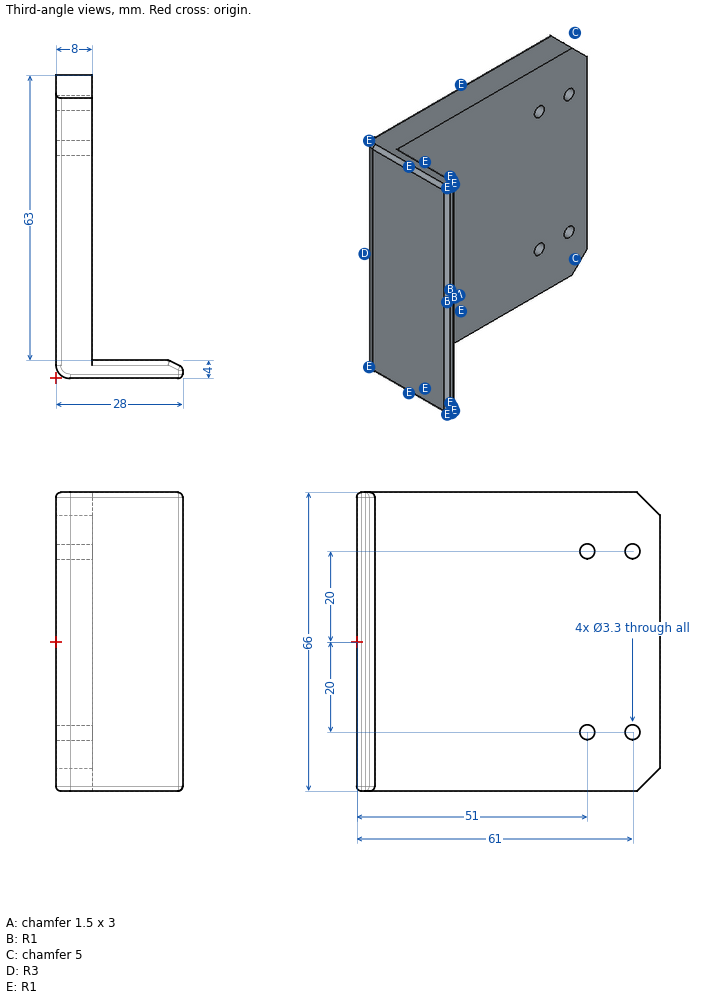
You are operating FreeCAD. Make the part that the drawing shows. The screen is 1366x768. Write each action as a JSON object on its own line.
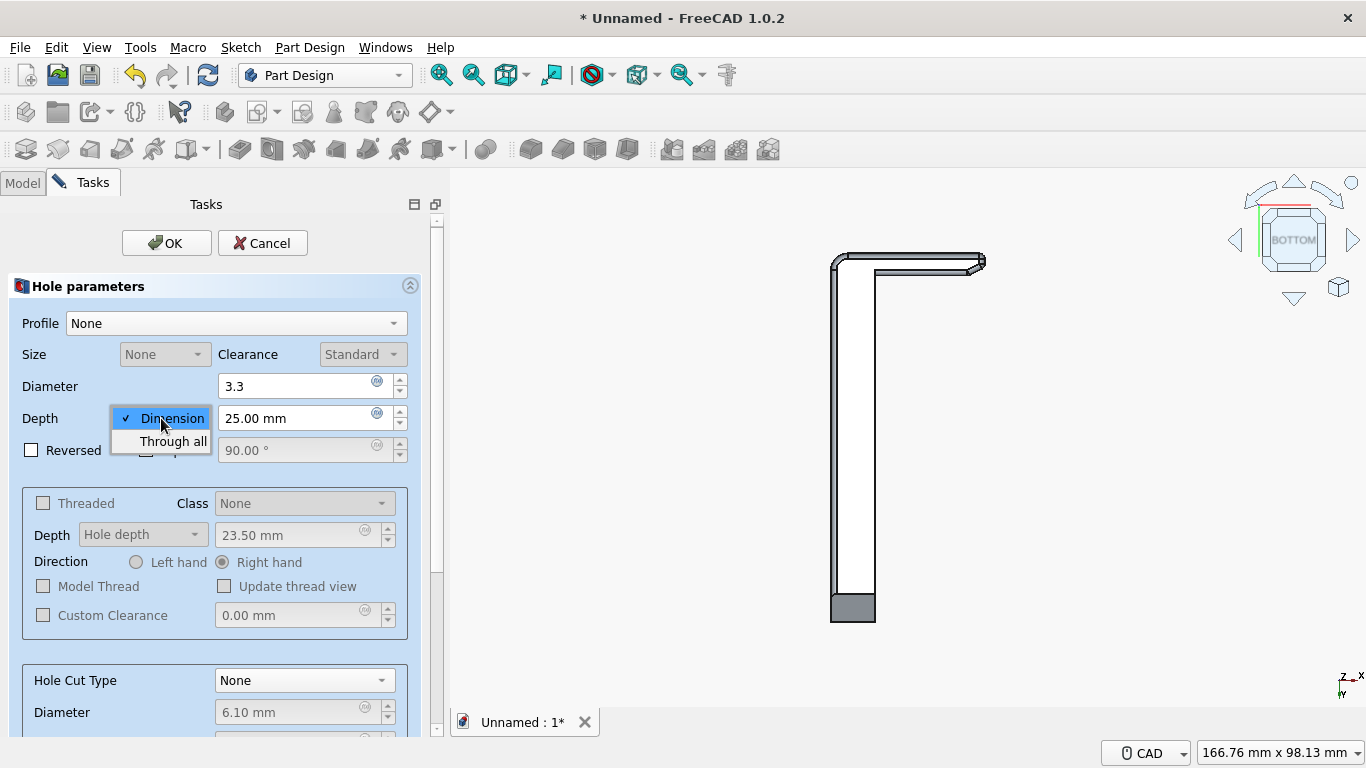
{"action": "left_click", "coordinate": [160, 442]}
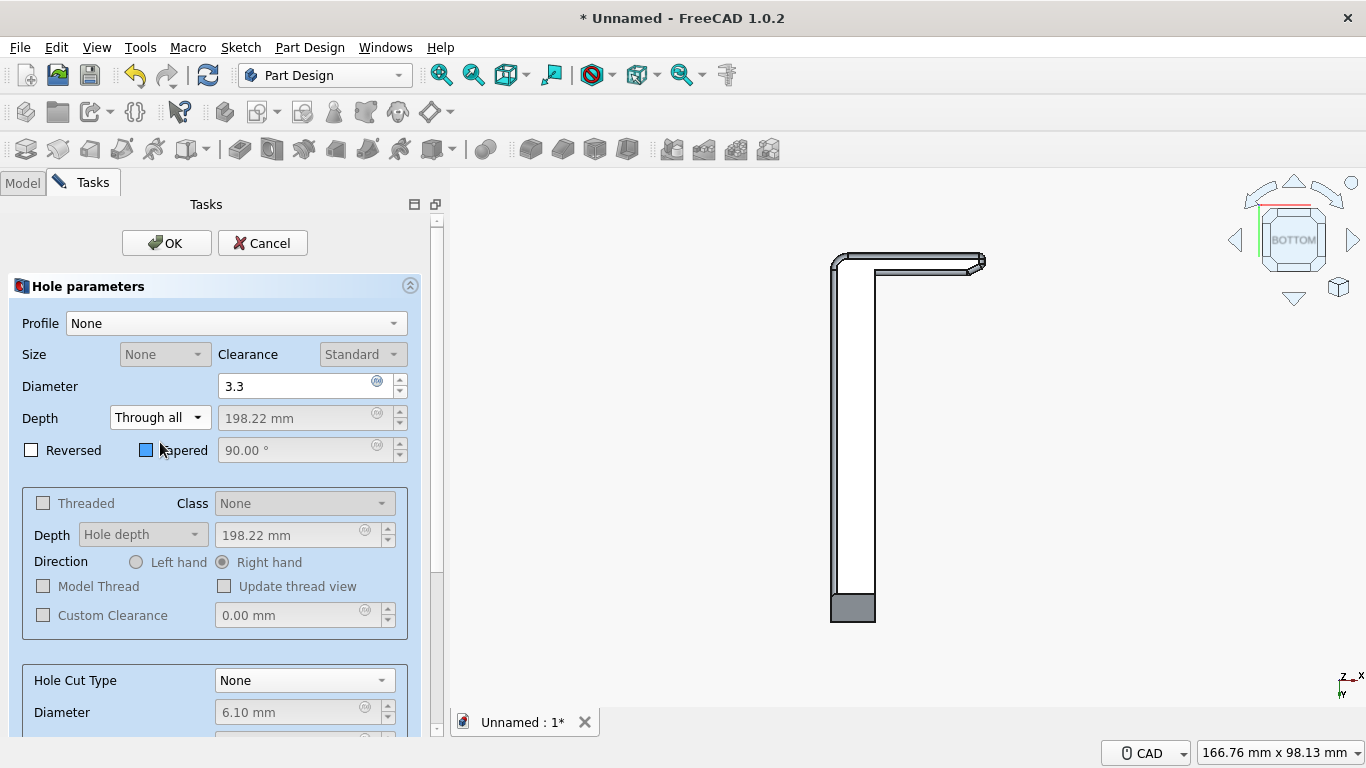
{"action": "left_click", "coordinate": [30, 450]}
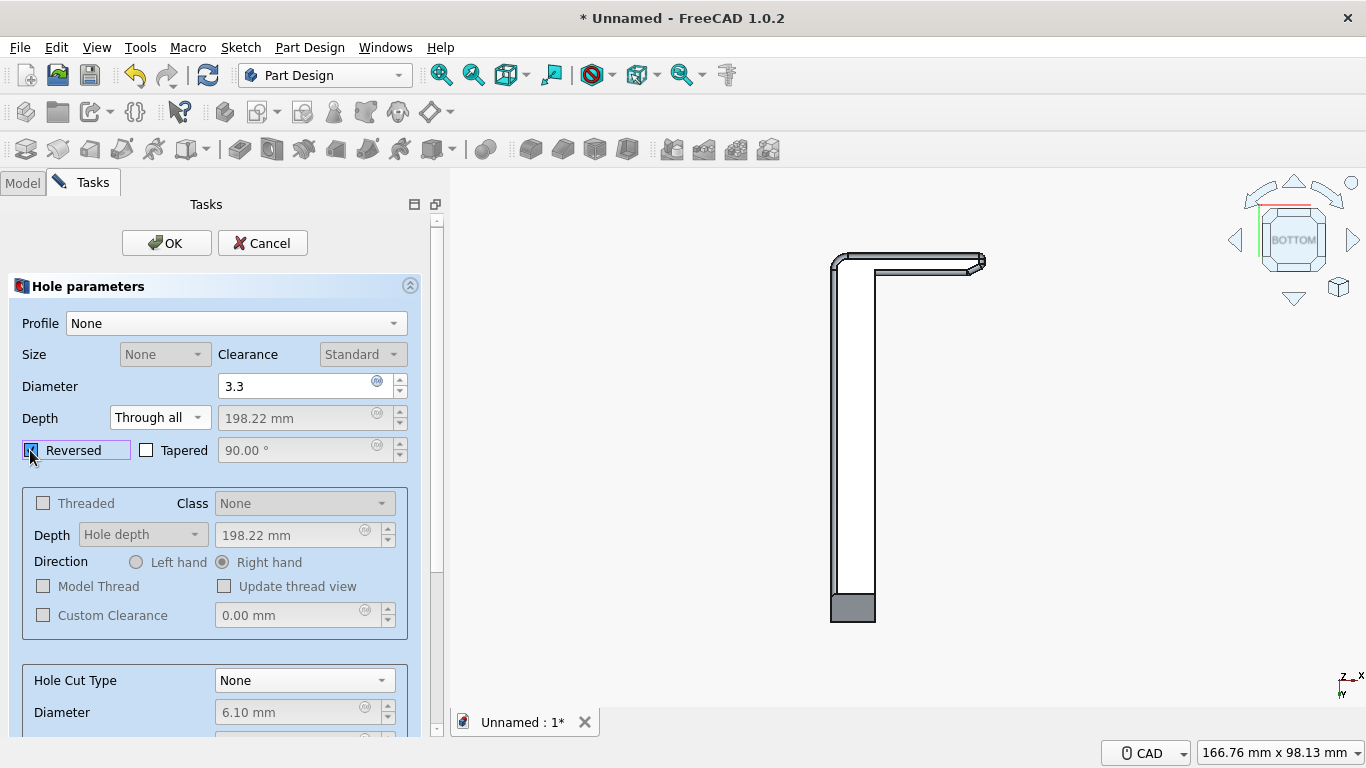
{"action": "left_click", "coordinate": [167, 243]}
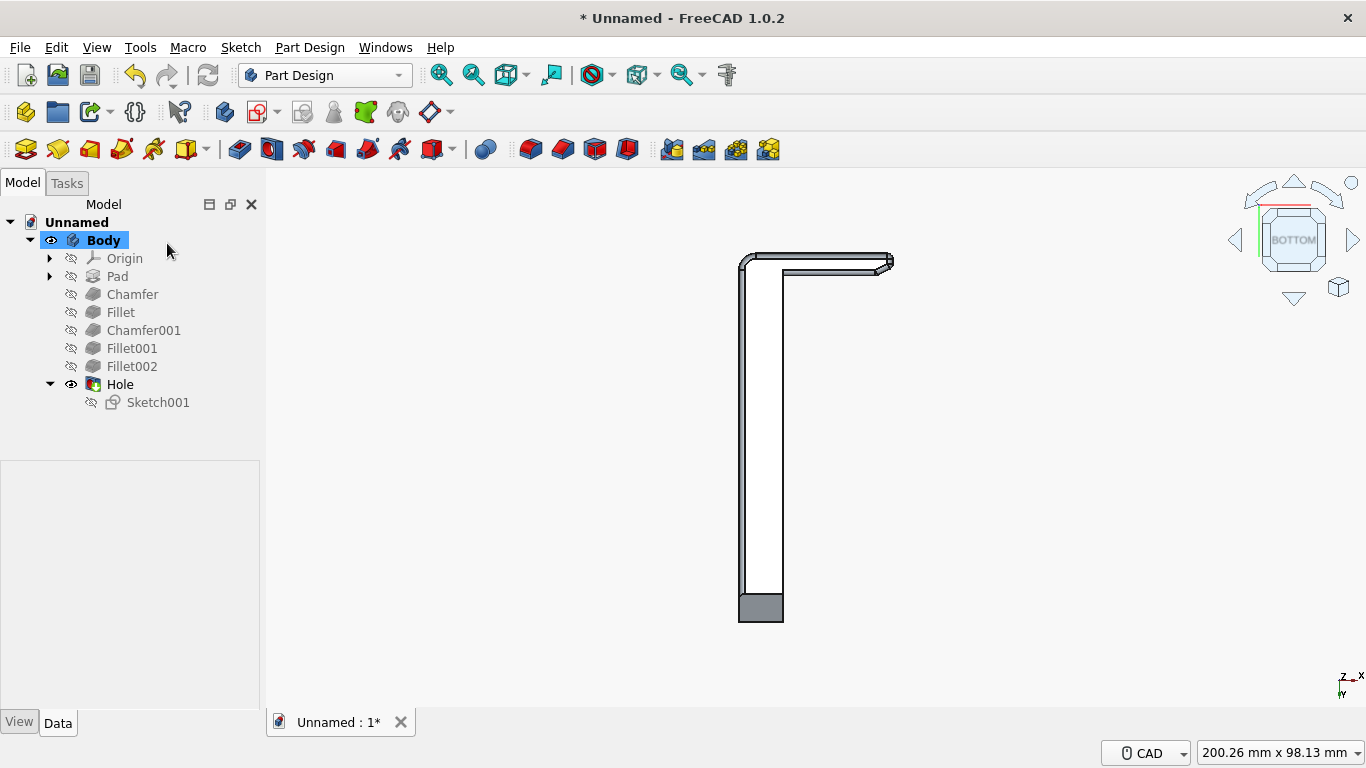
{"action": "key", "text": "0"}